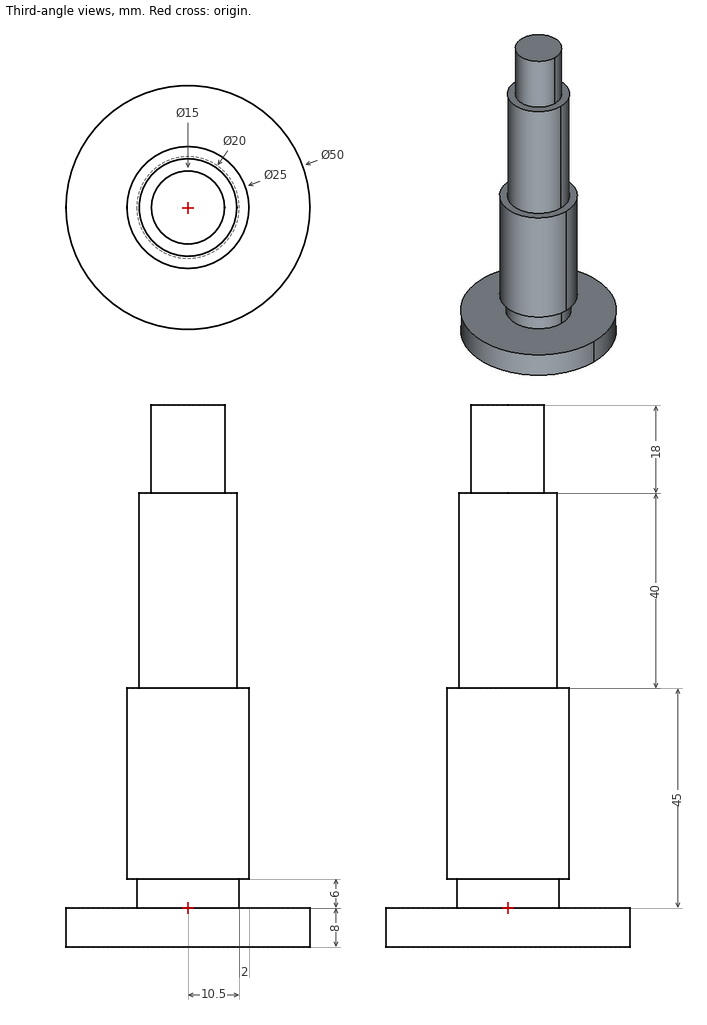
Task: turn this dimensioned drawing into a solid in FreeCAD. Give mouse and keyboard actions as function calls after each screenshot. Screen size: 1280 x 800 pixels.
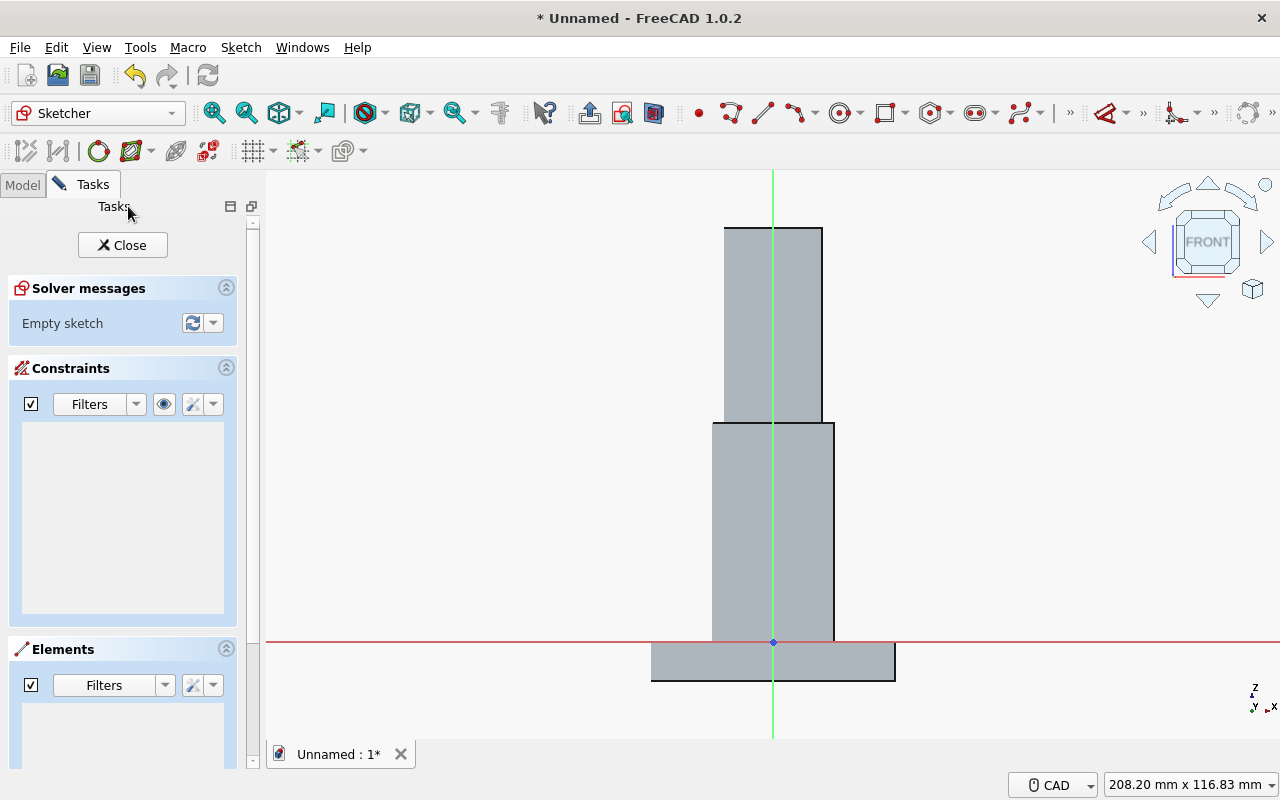
scroll(816, 649, up, 11)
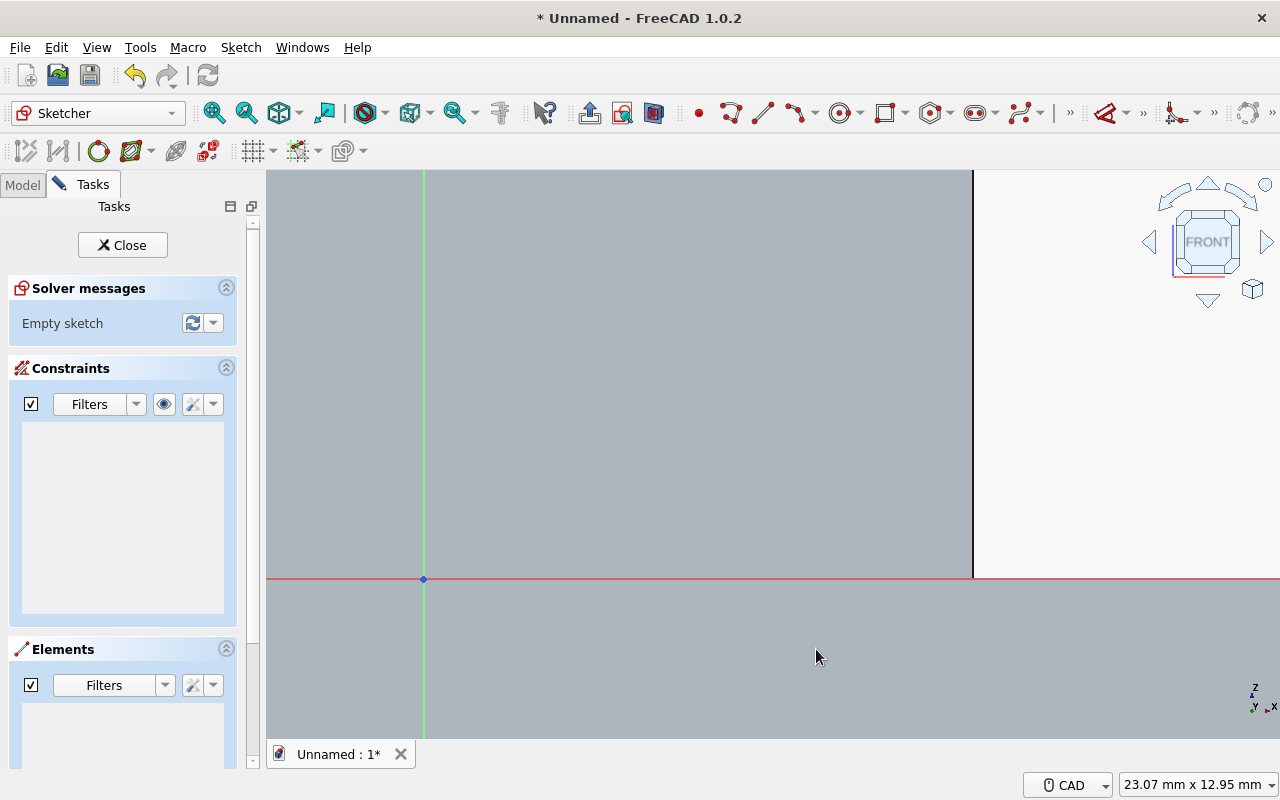
key(g)
key(r)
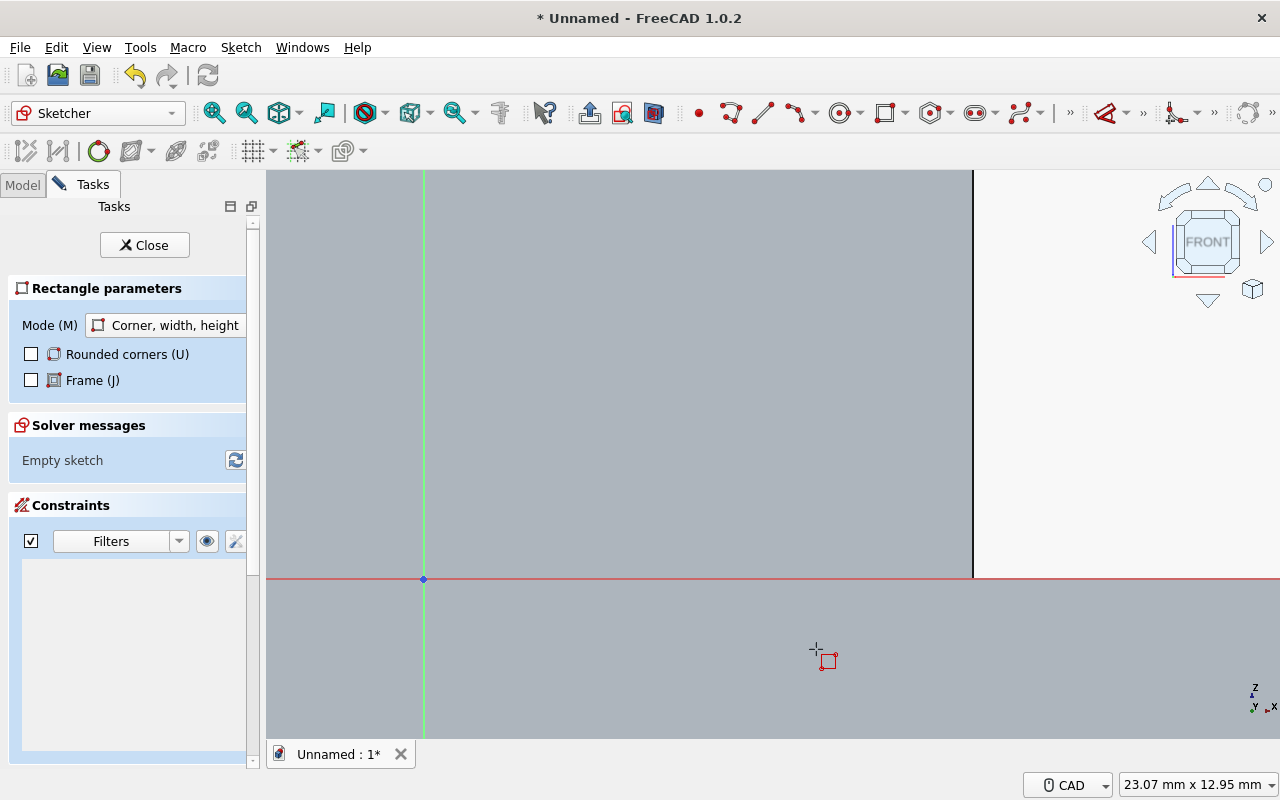
click(885, 315)
click(973, 579)
key(Escape)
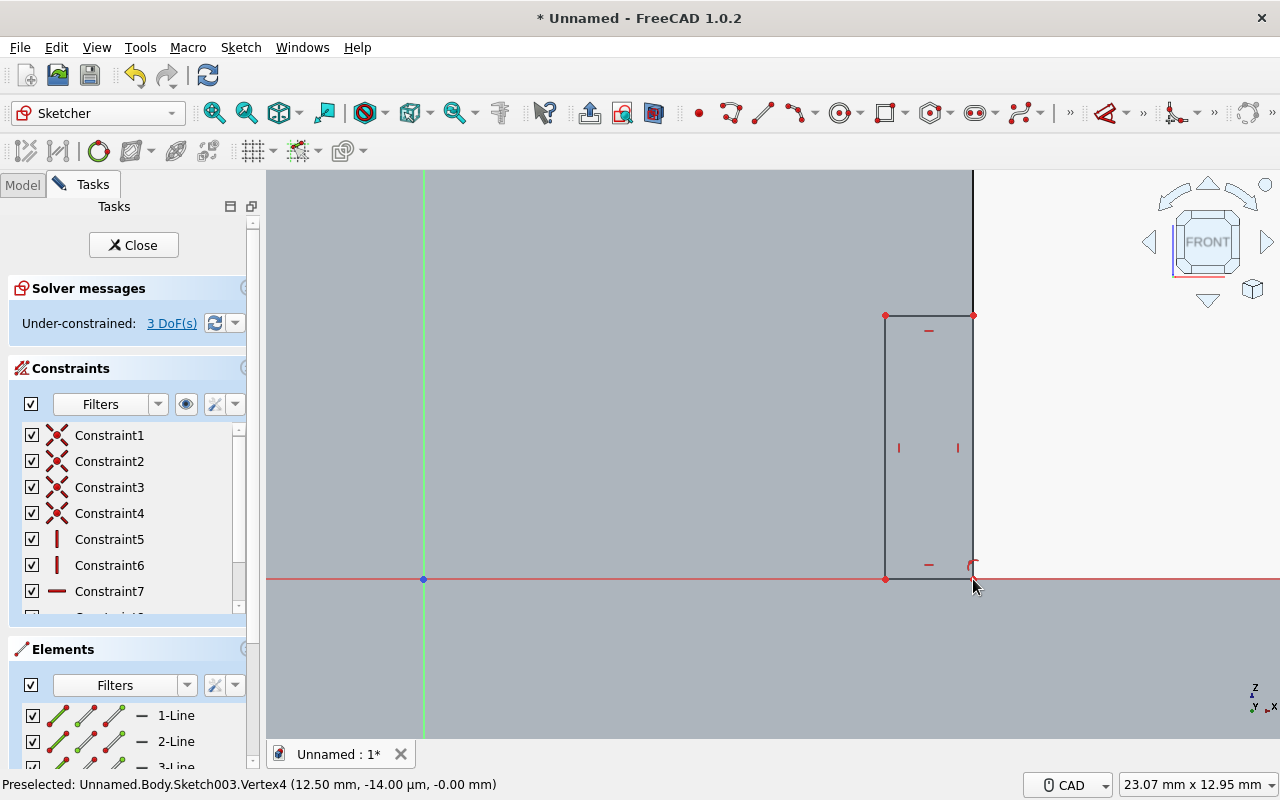
click(885, 395)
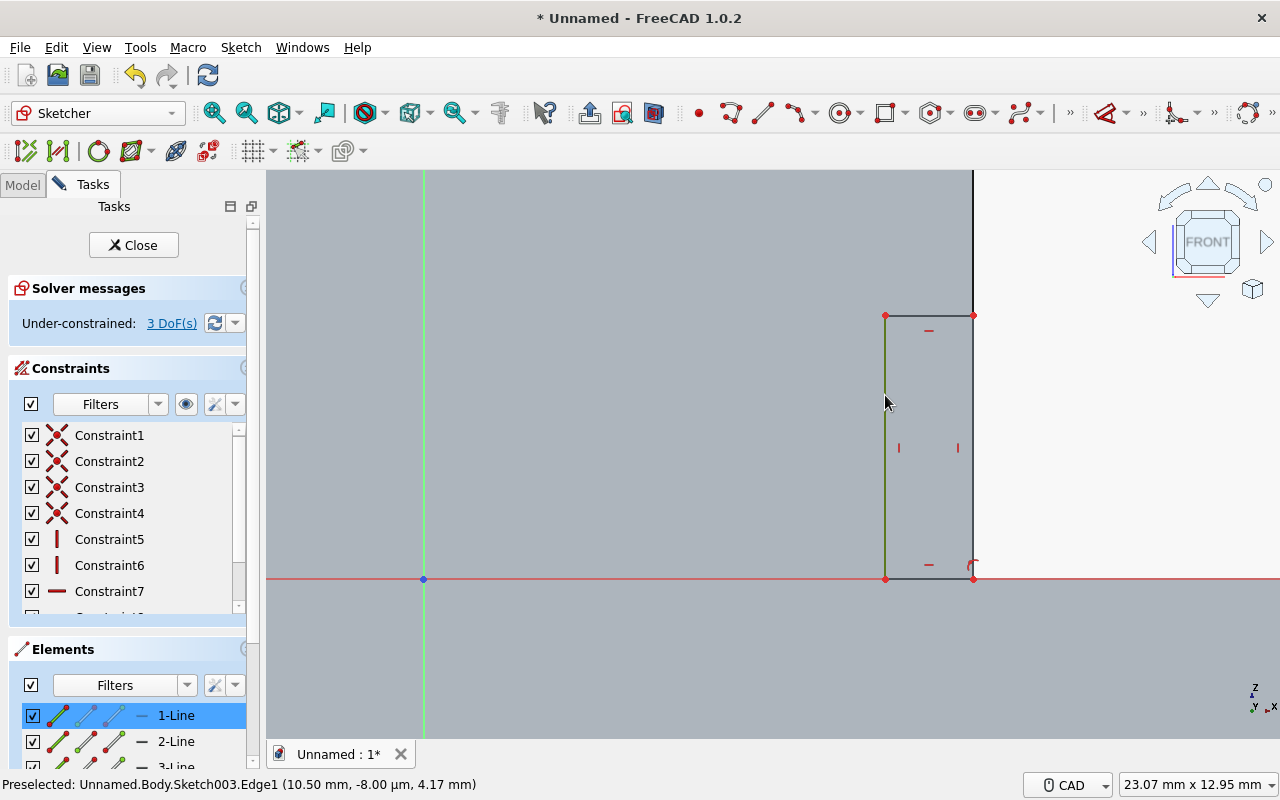
key(i)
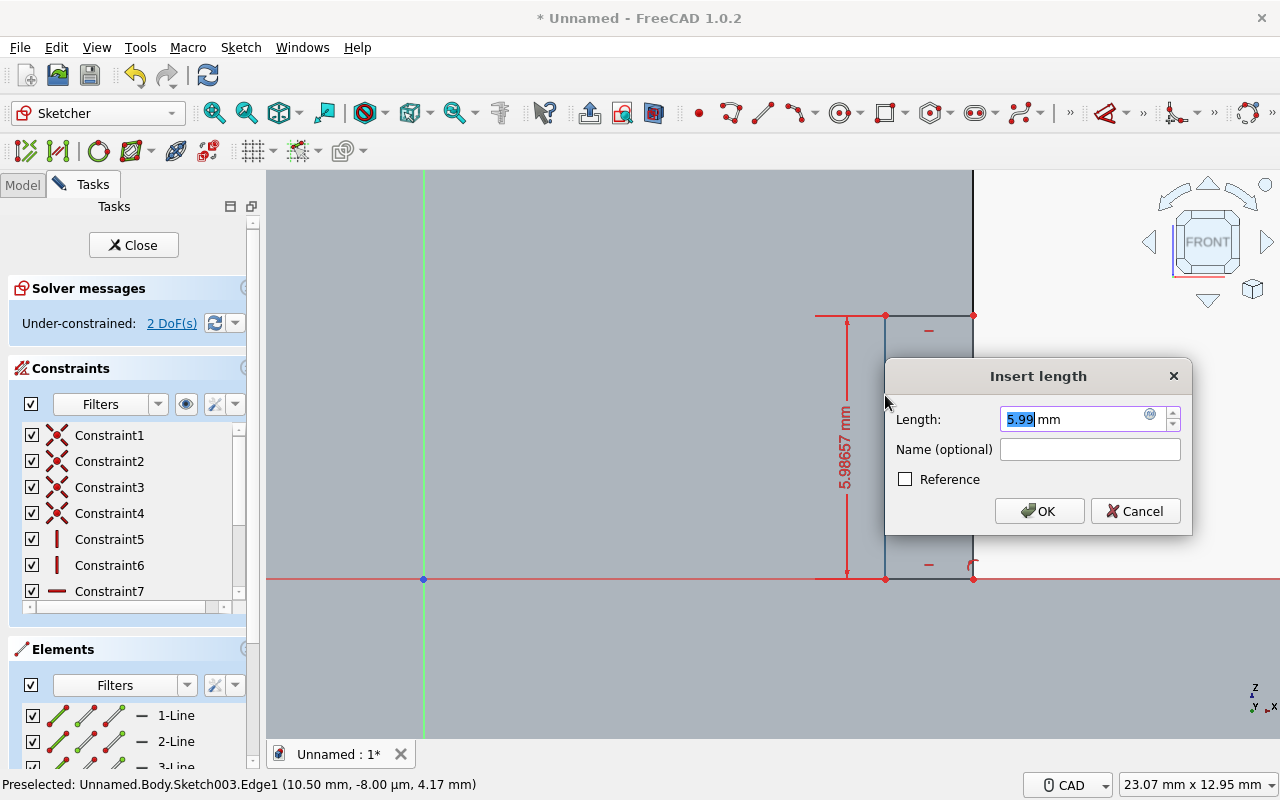
text(6)
key(Return)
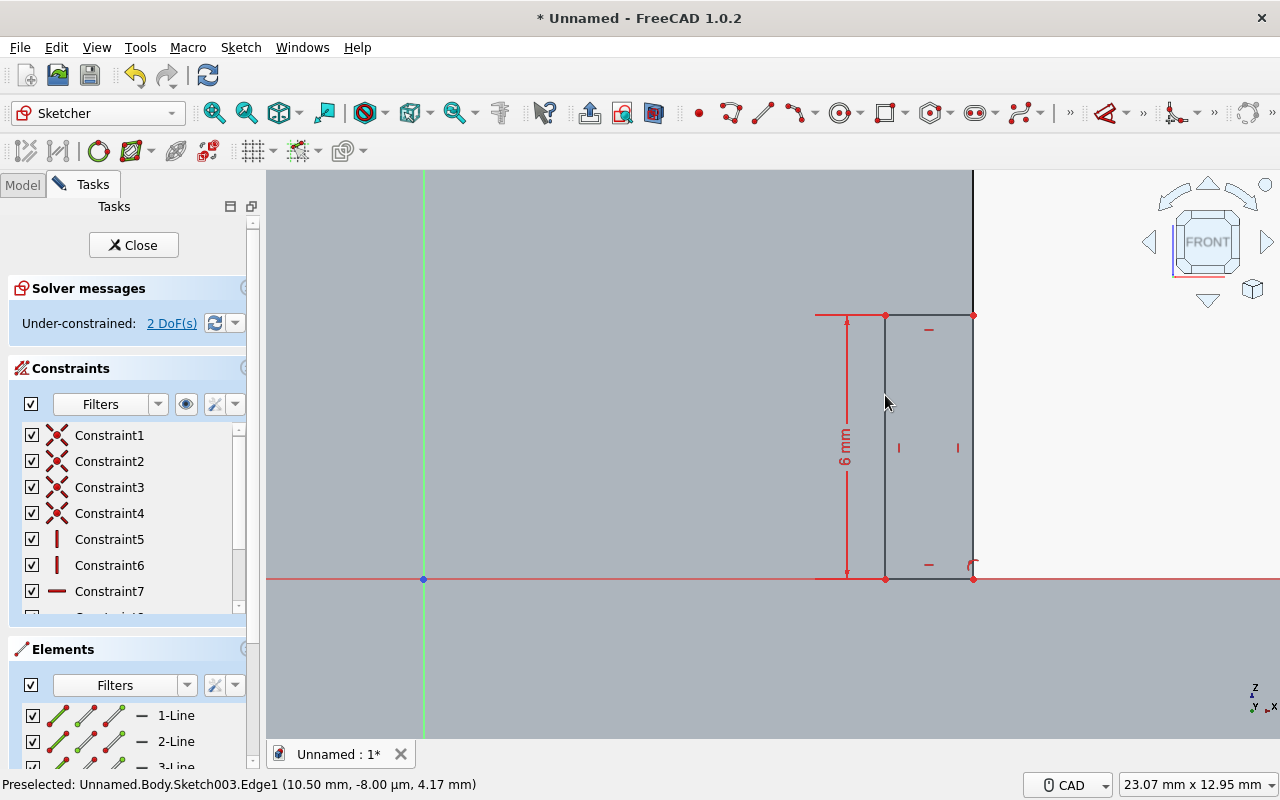
click(911, 579)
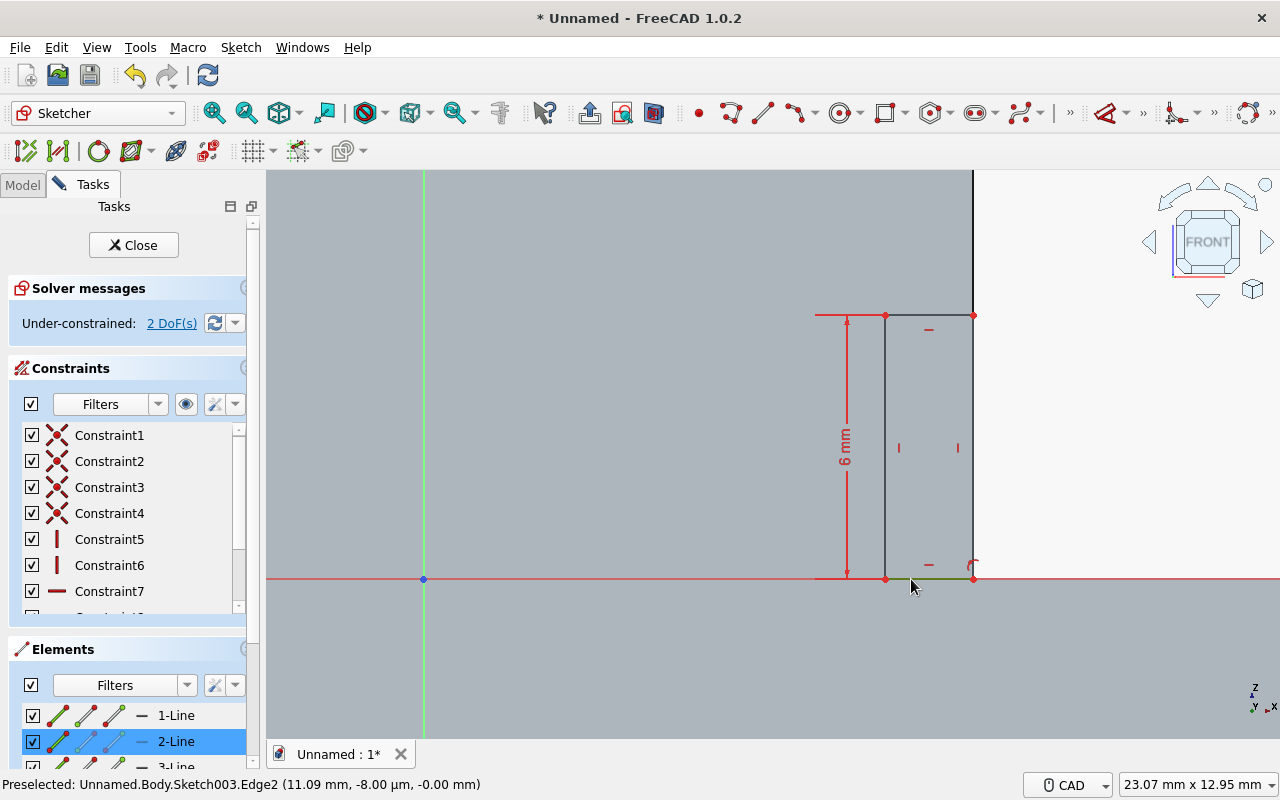
key(l)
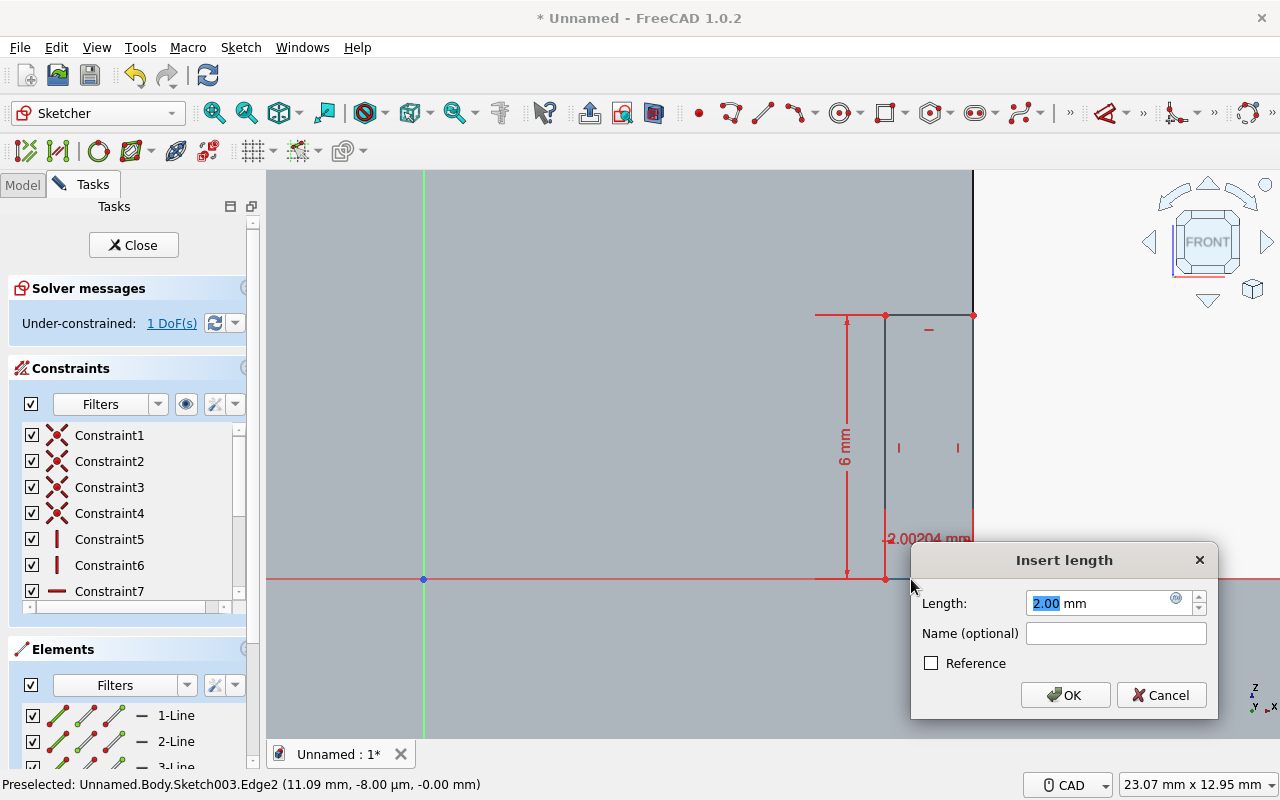
text(2)
key(Return)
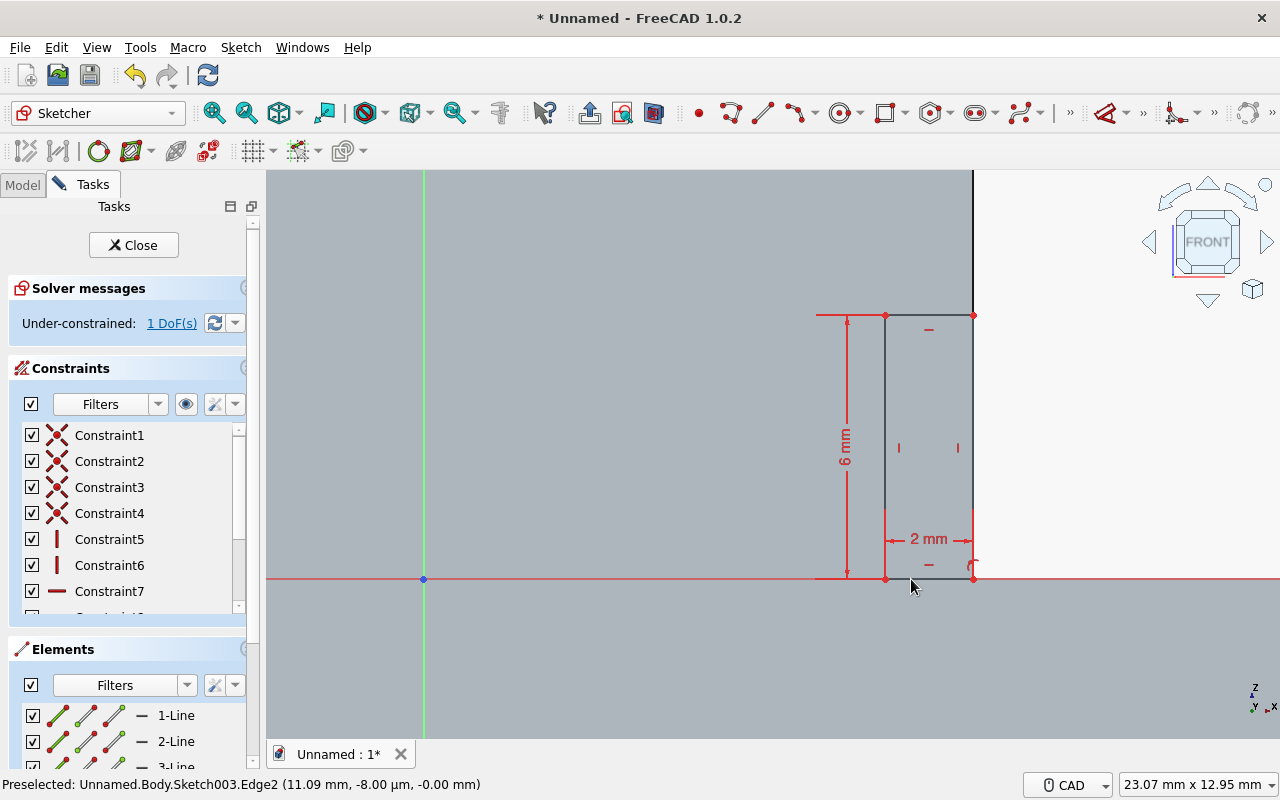
click(885, 315)